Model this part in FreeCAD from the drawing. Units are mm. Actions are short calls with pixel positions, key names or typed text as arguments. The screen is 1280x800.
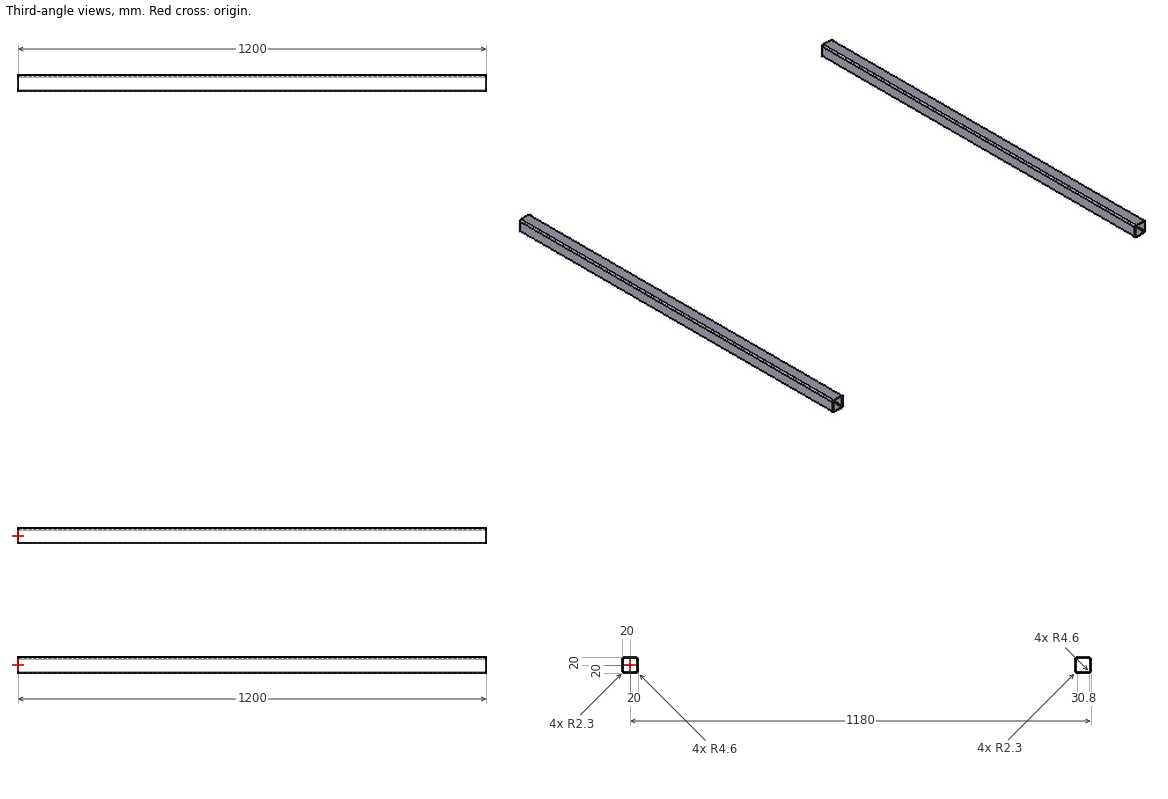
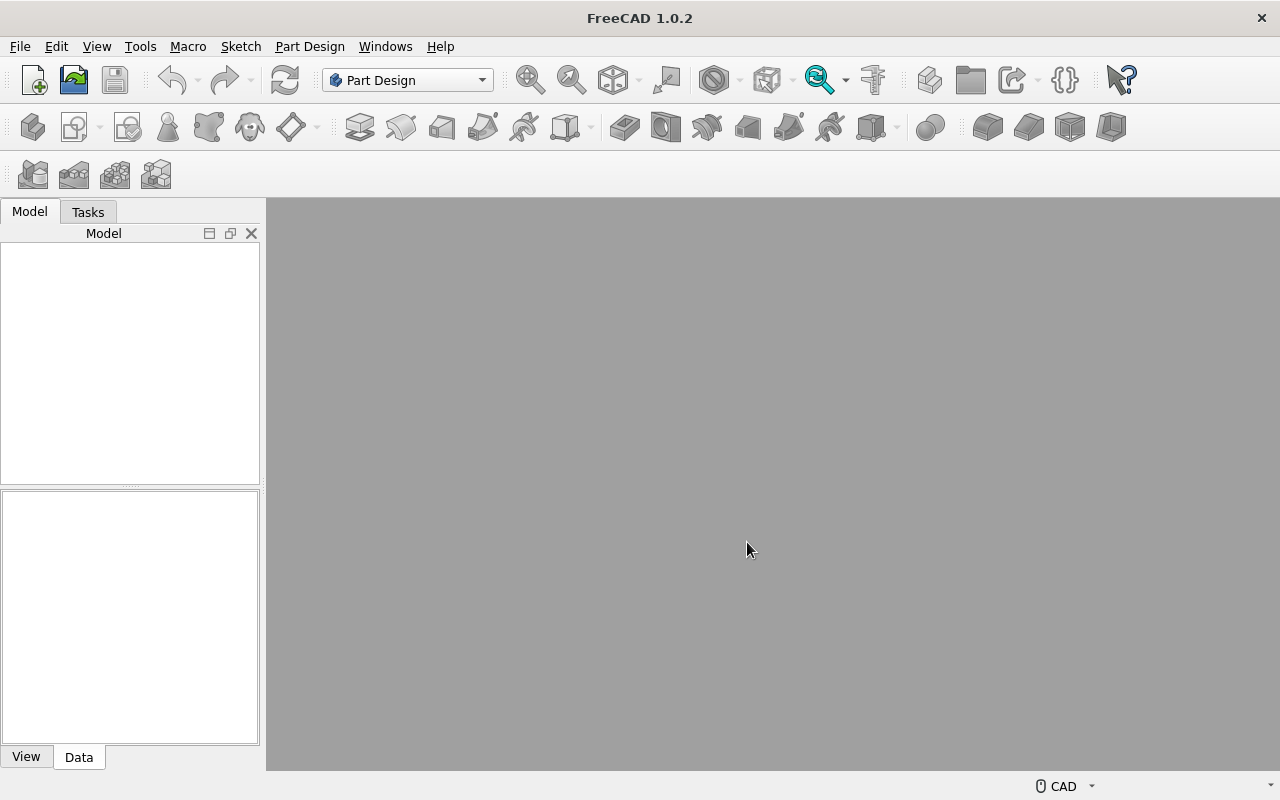
key(ctrl+n)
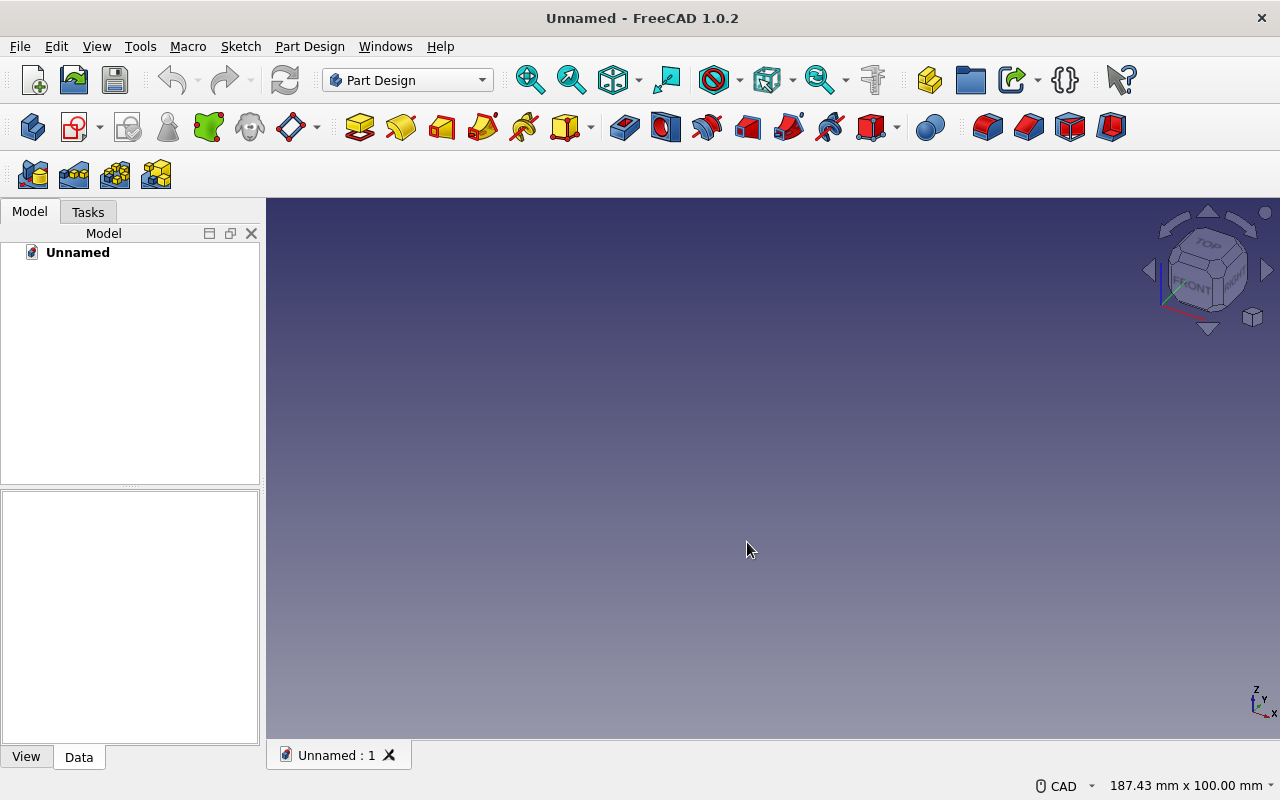
click(74, 128)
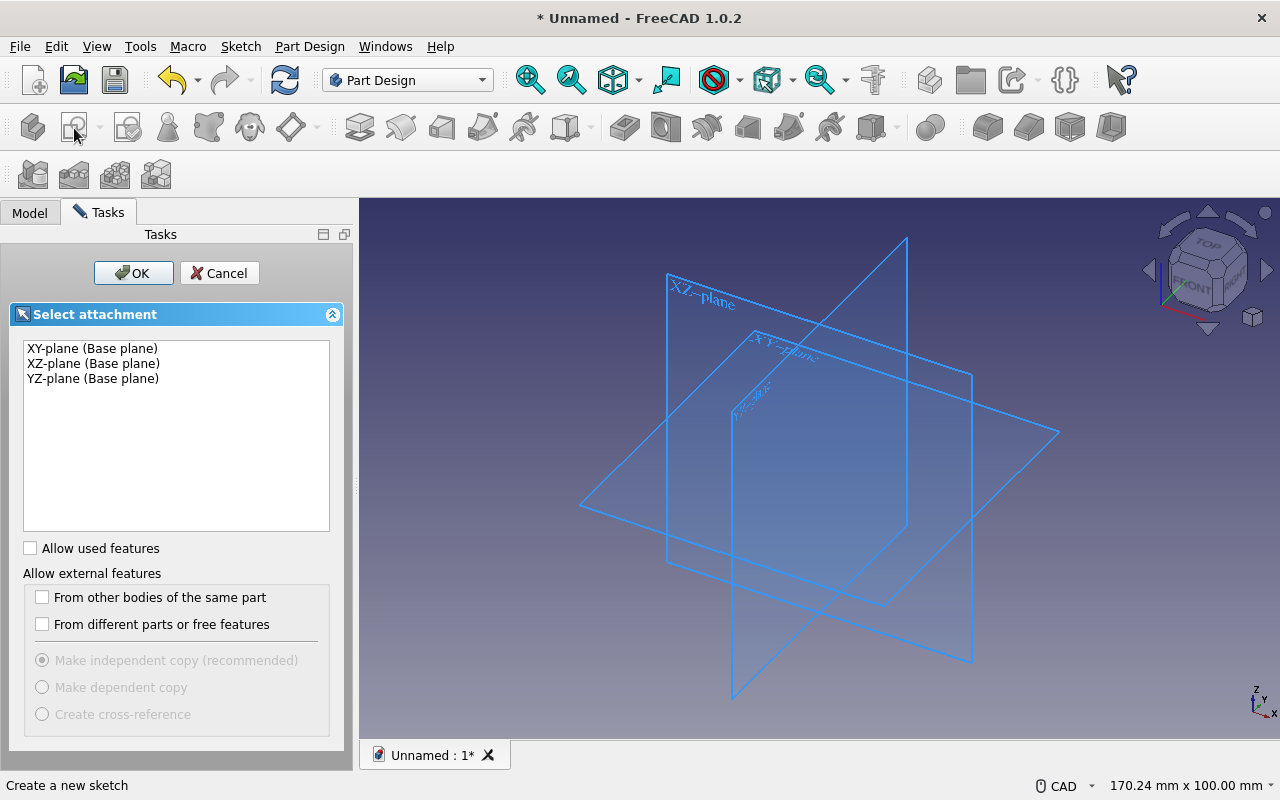
click(84, 378)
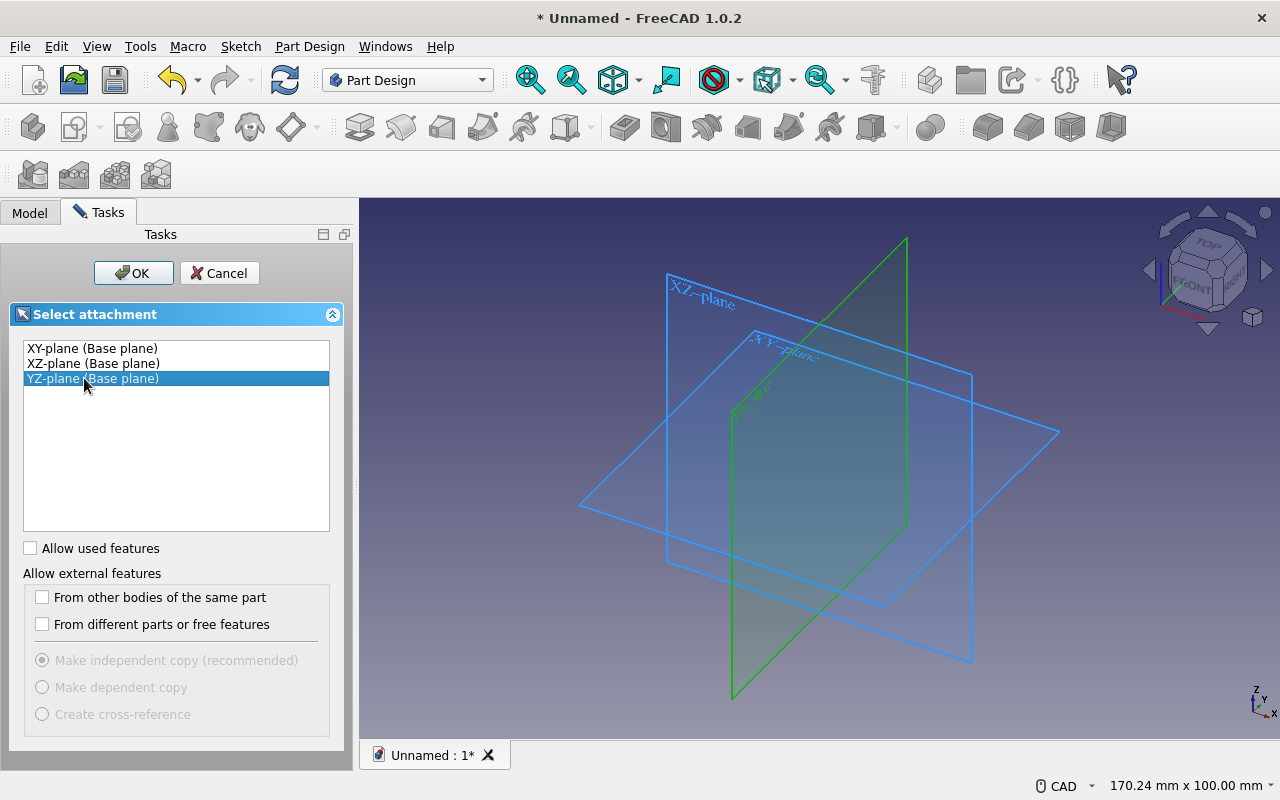
click(134, 273)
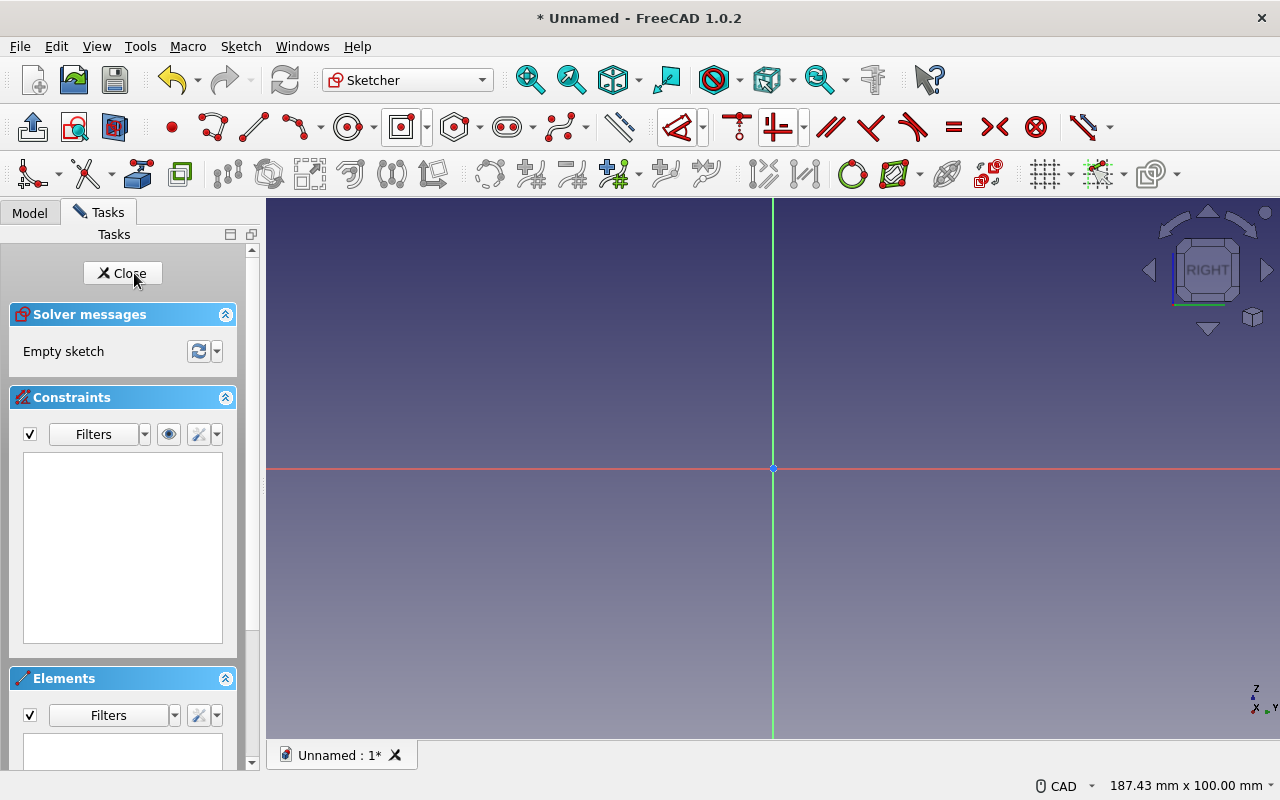
scroll(912, 469, up, 2)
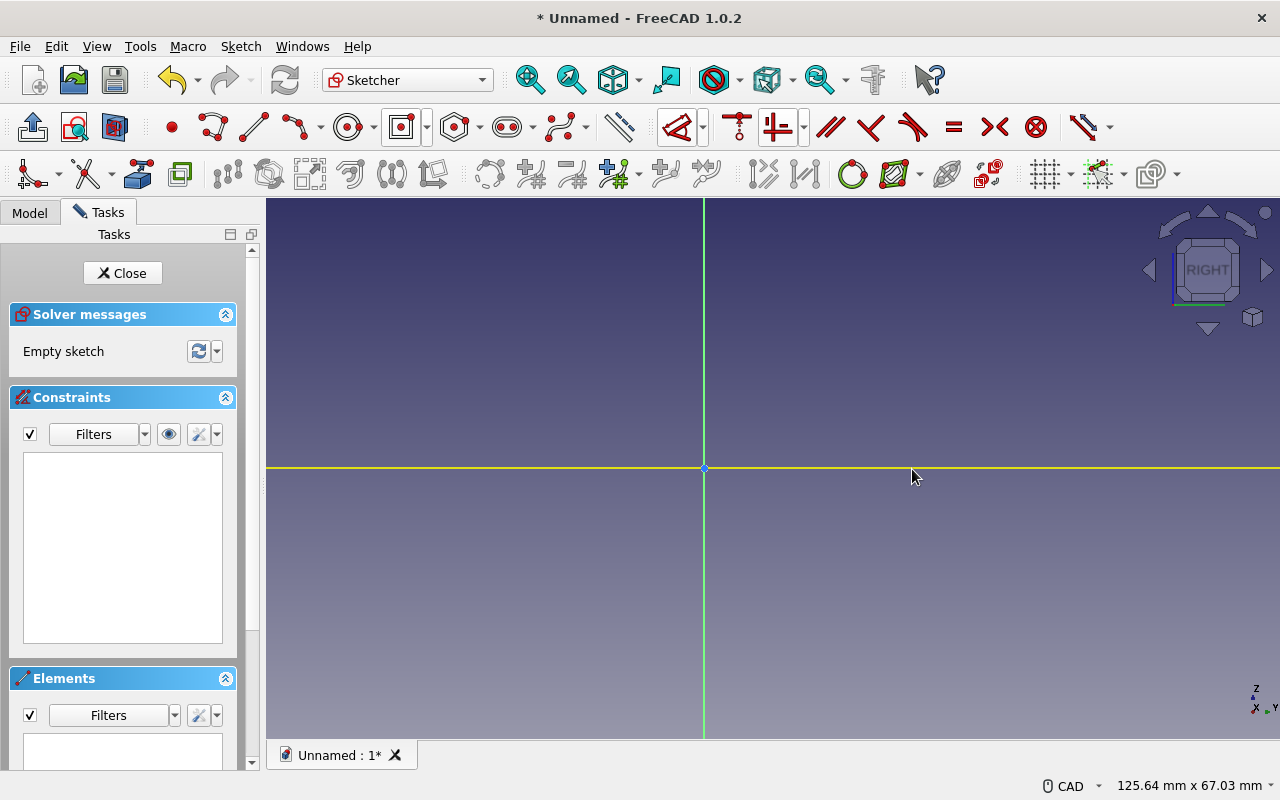
key(g)
key(l)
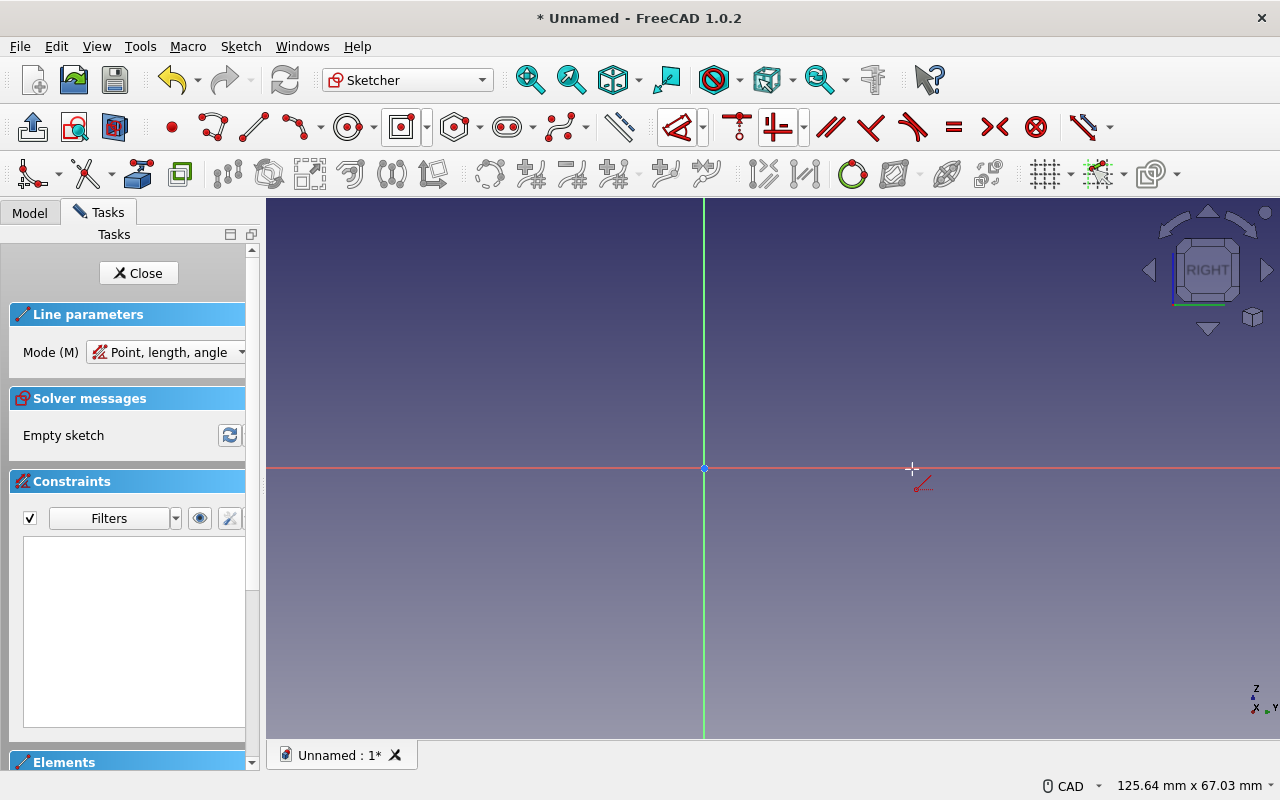
click(580, 629)
click(829, 629)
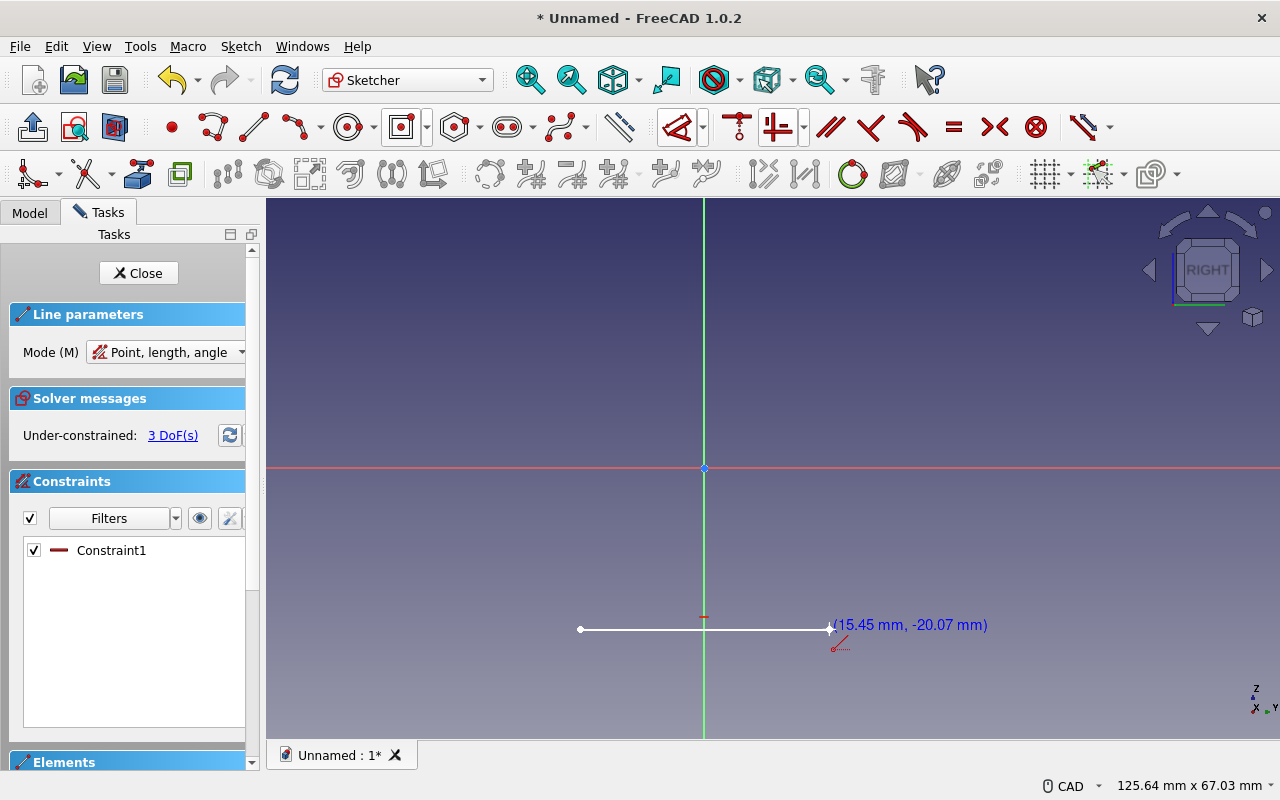
click(866, 592)
click(866, 344)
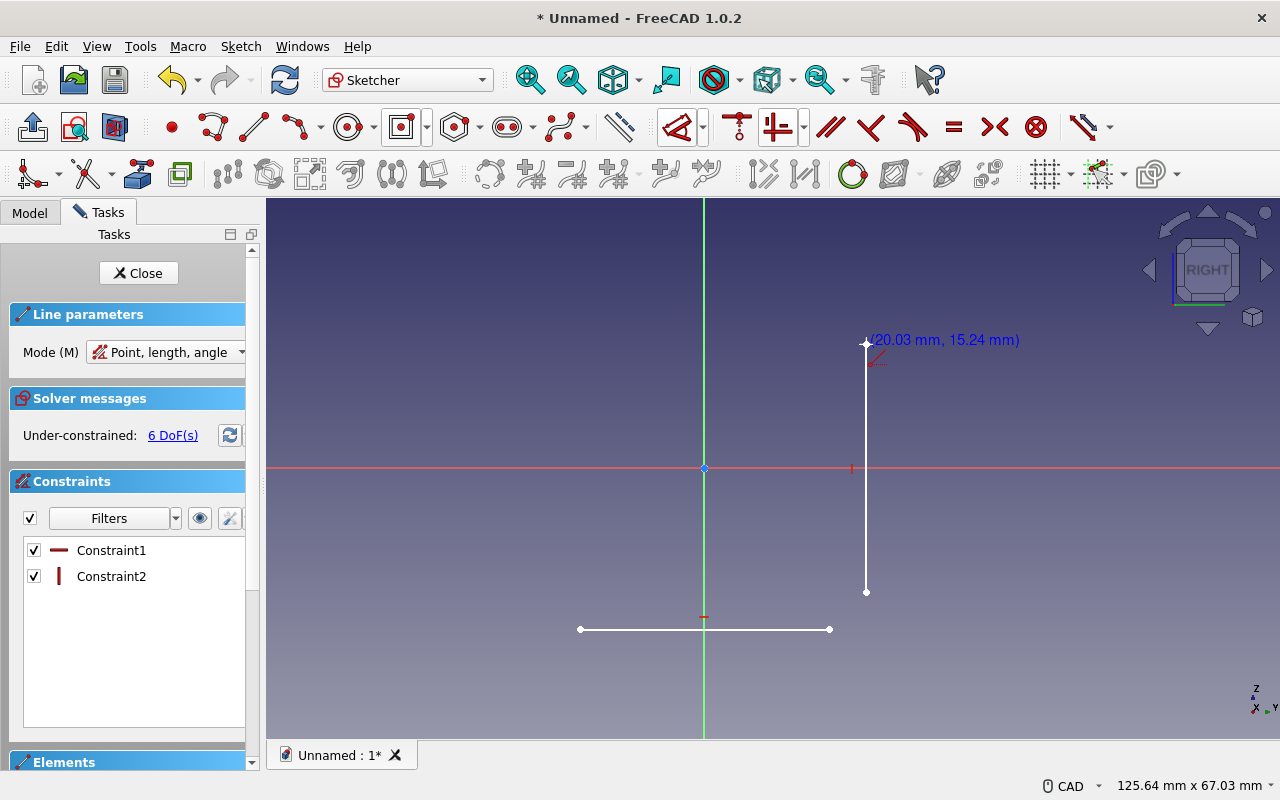
click(829, 307)
click(580, 307)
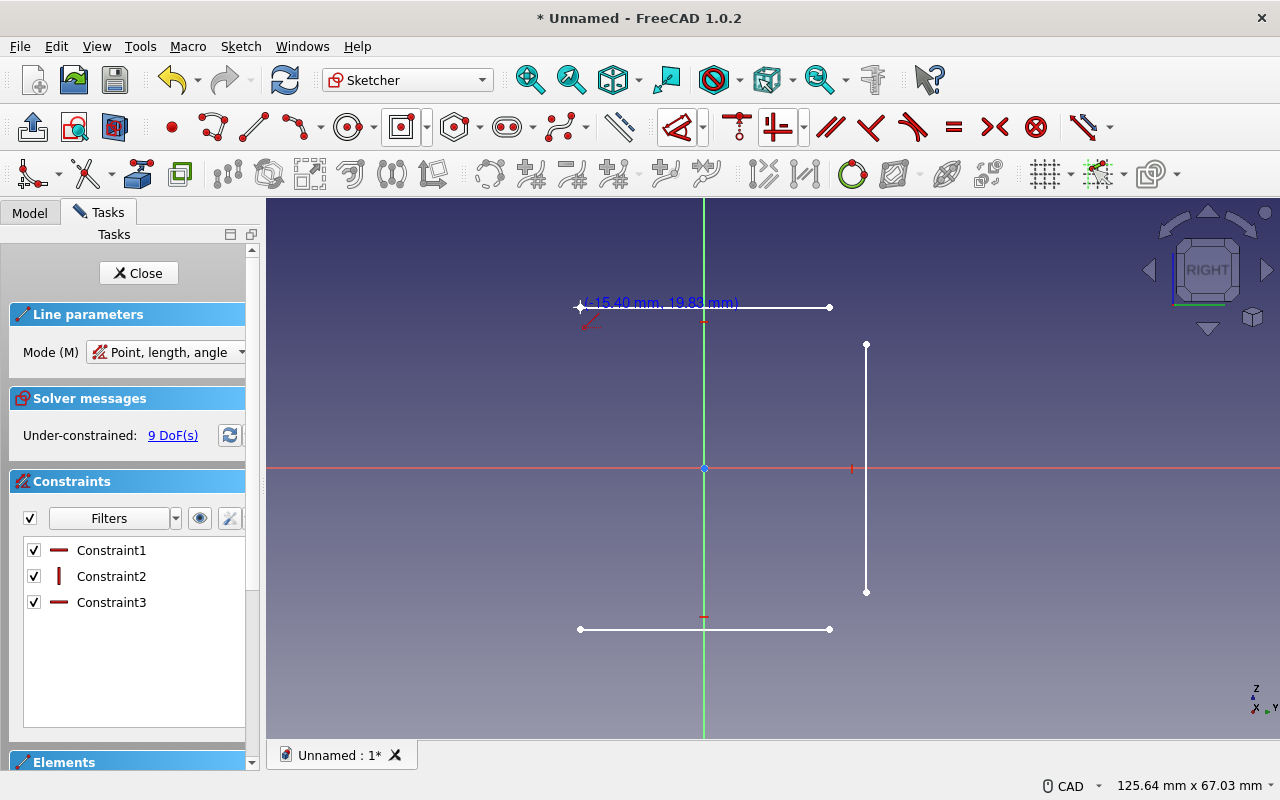
click(543, 344)
click(543, 592)